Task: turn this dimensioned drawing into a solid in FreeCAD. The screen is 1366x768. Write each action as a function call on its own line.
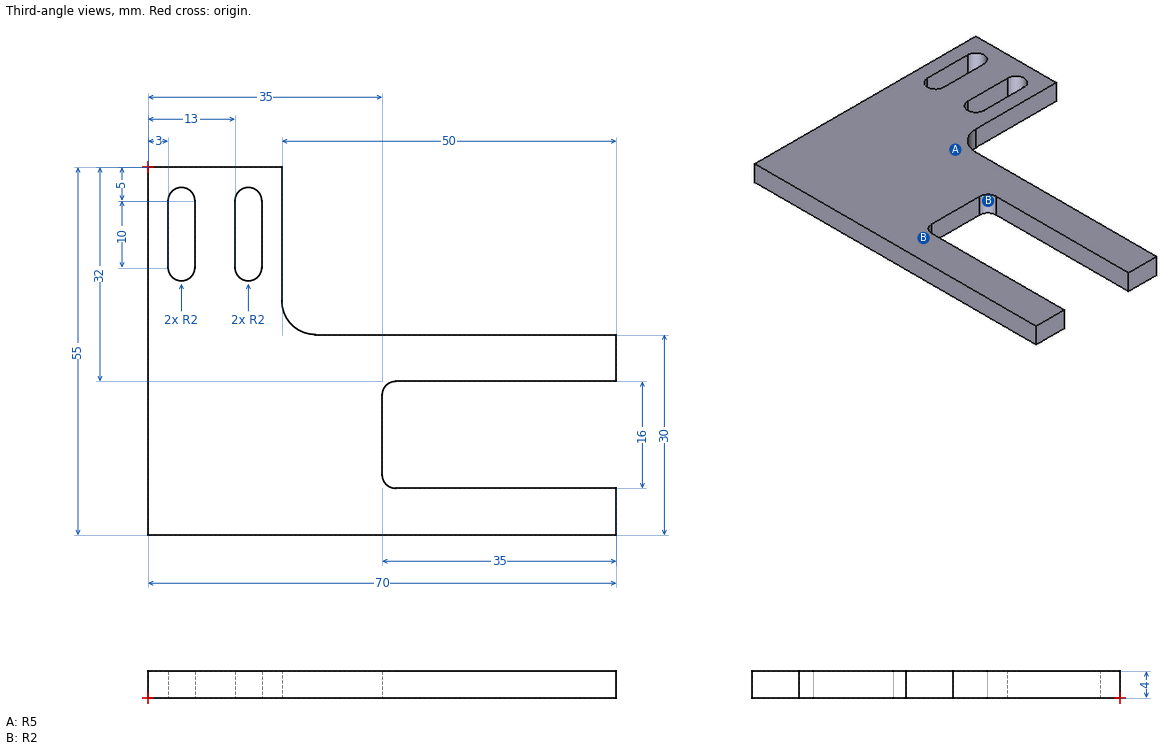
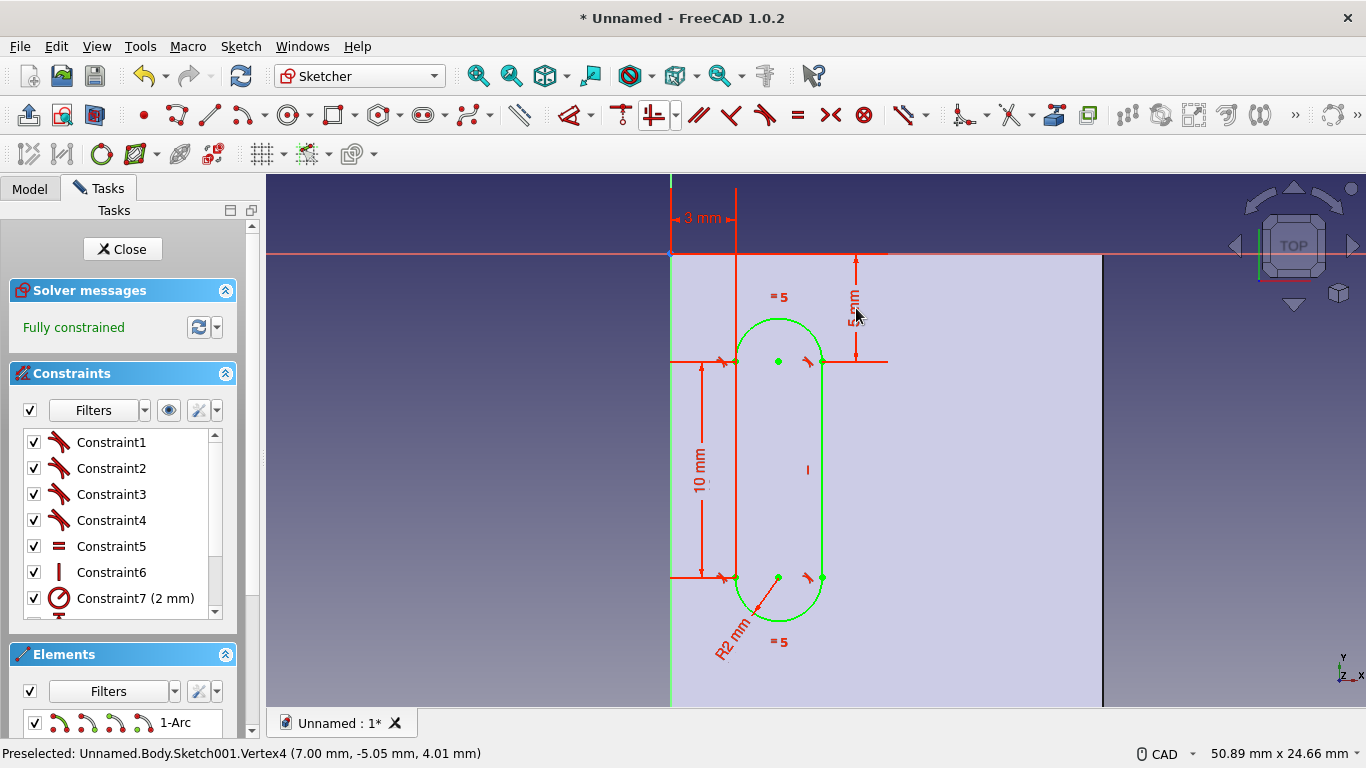
click(123, 249)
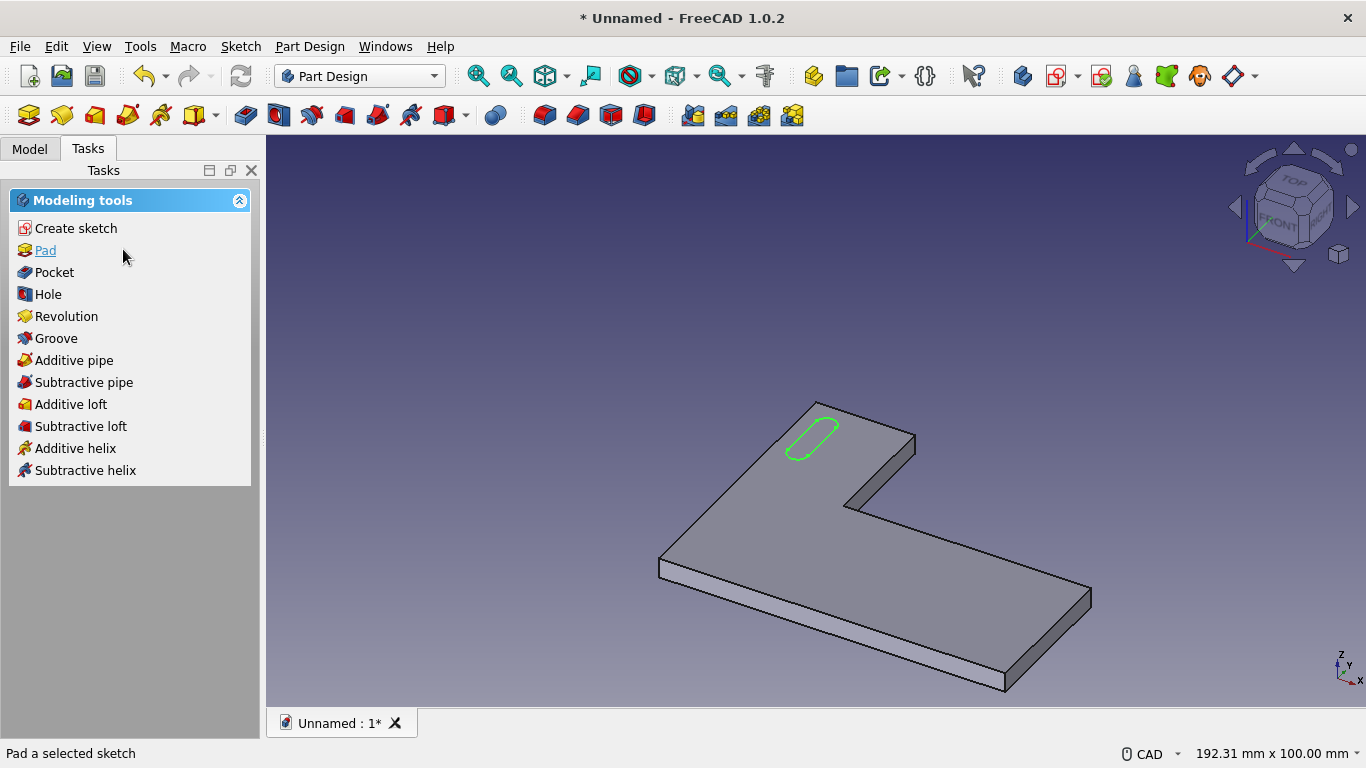
click(246, 116)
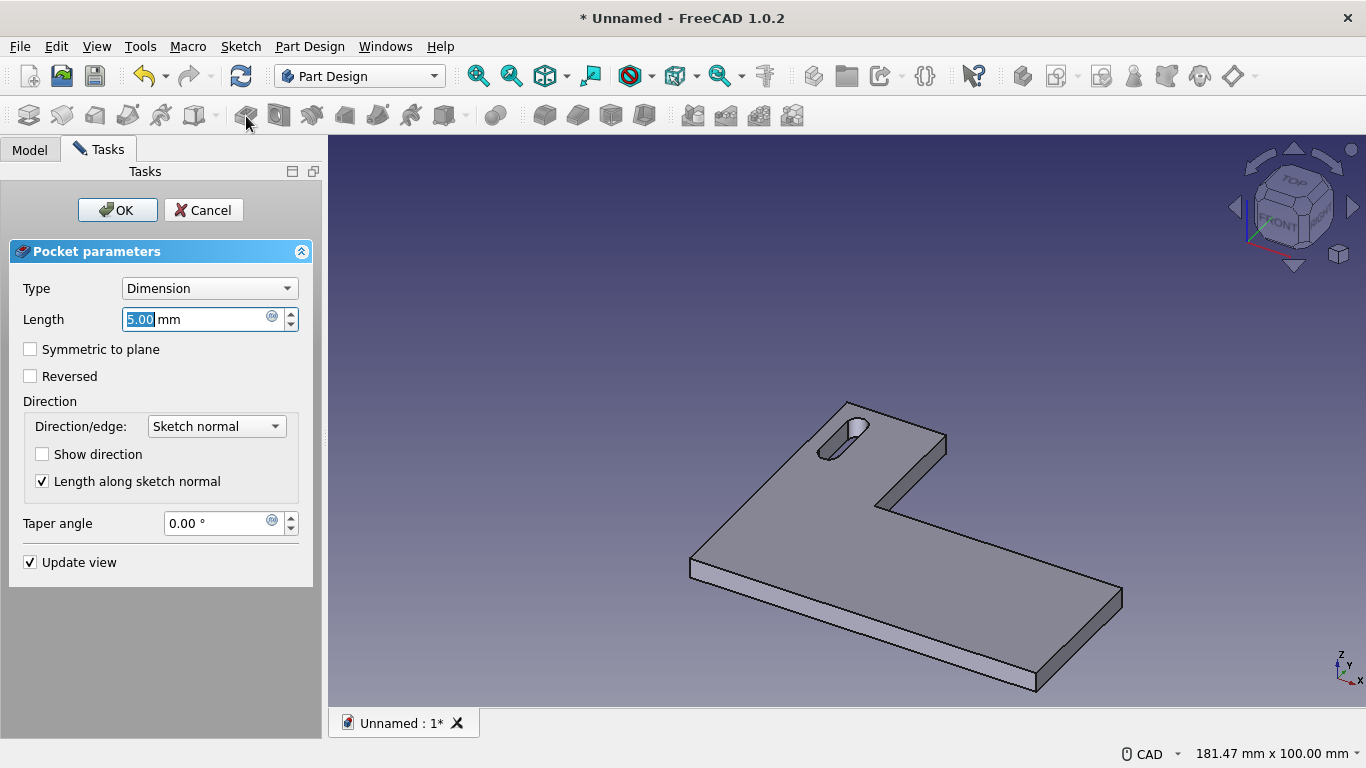
click(210, 288)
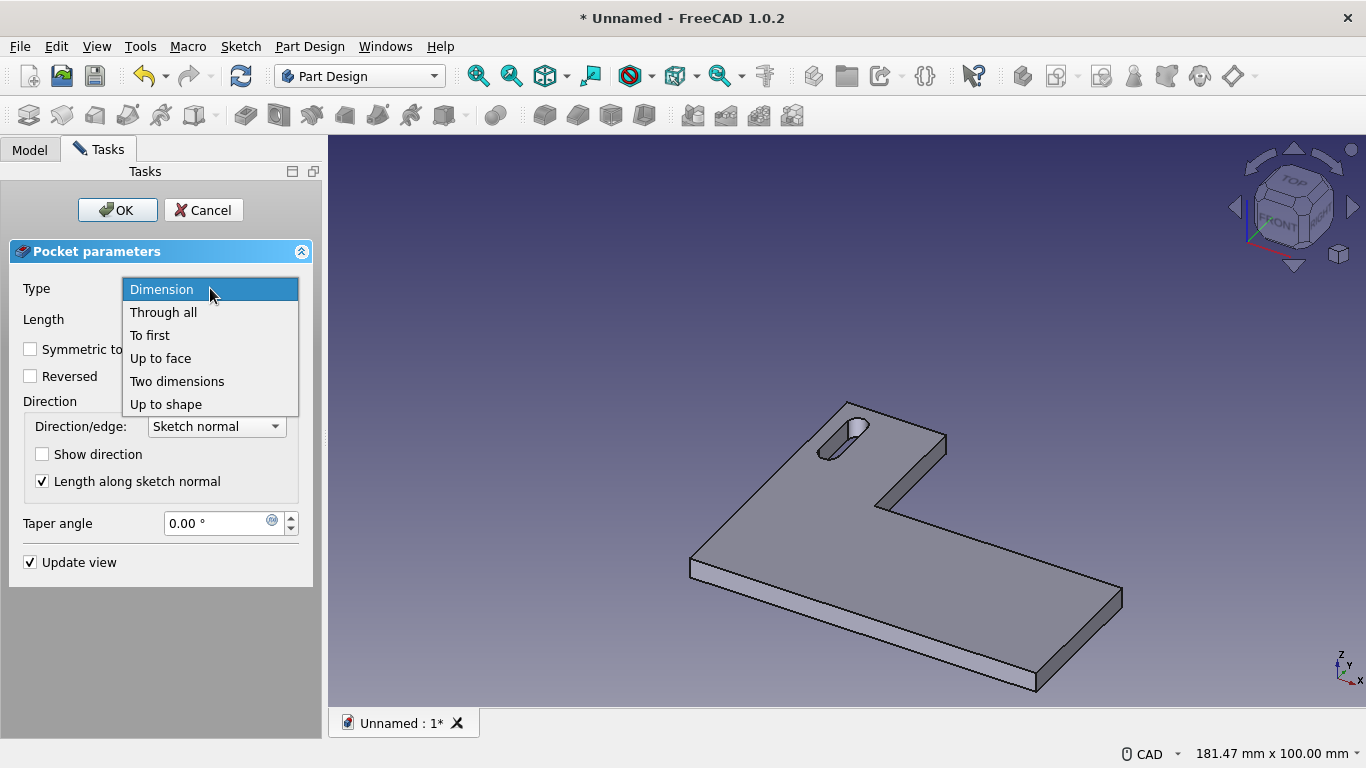
click(208, 336)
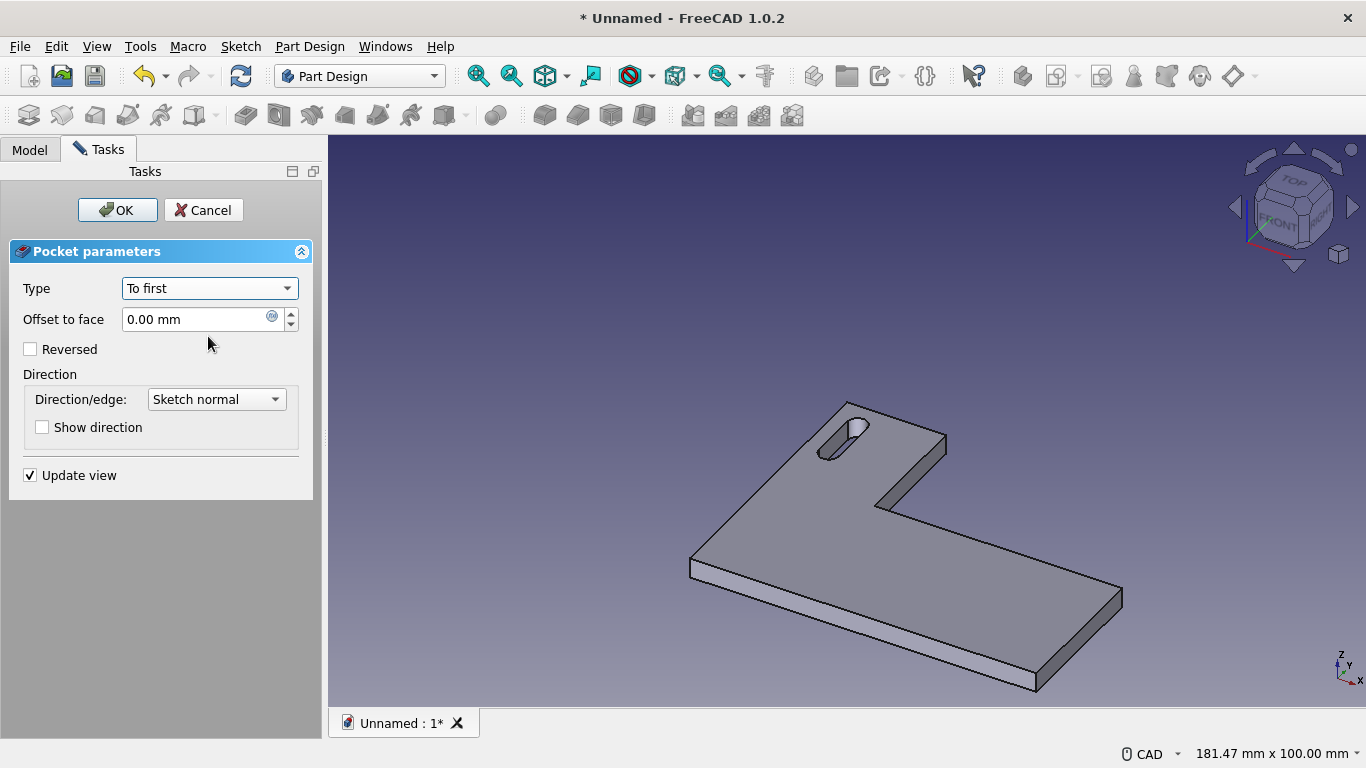
click(118, 210)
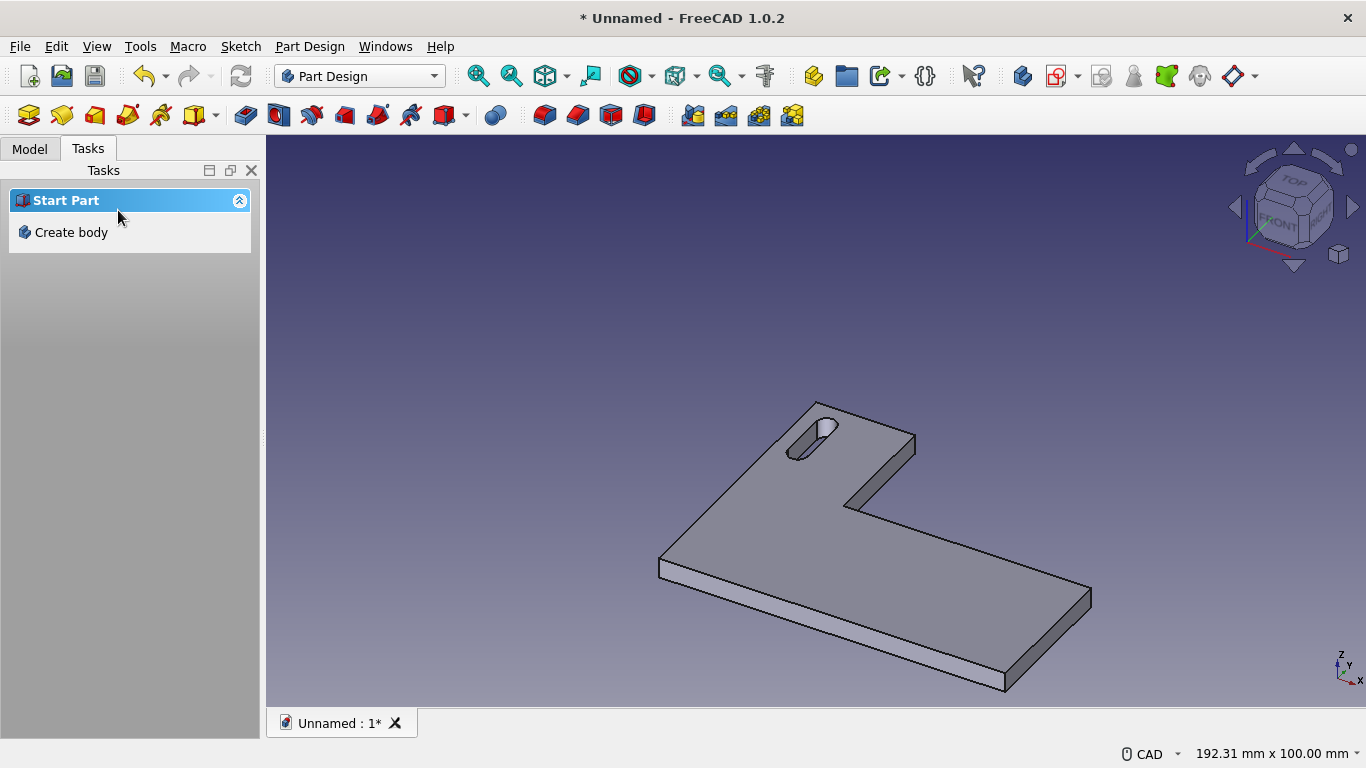
click(965, 614)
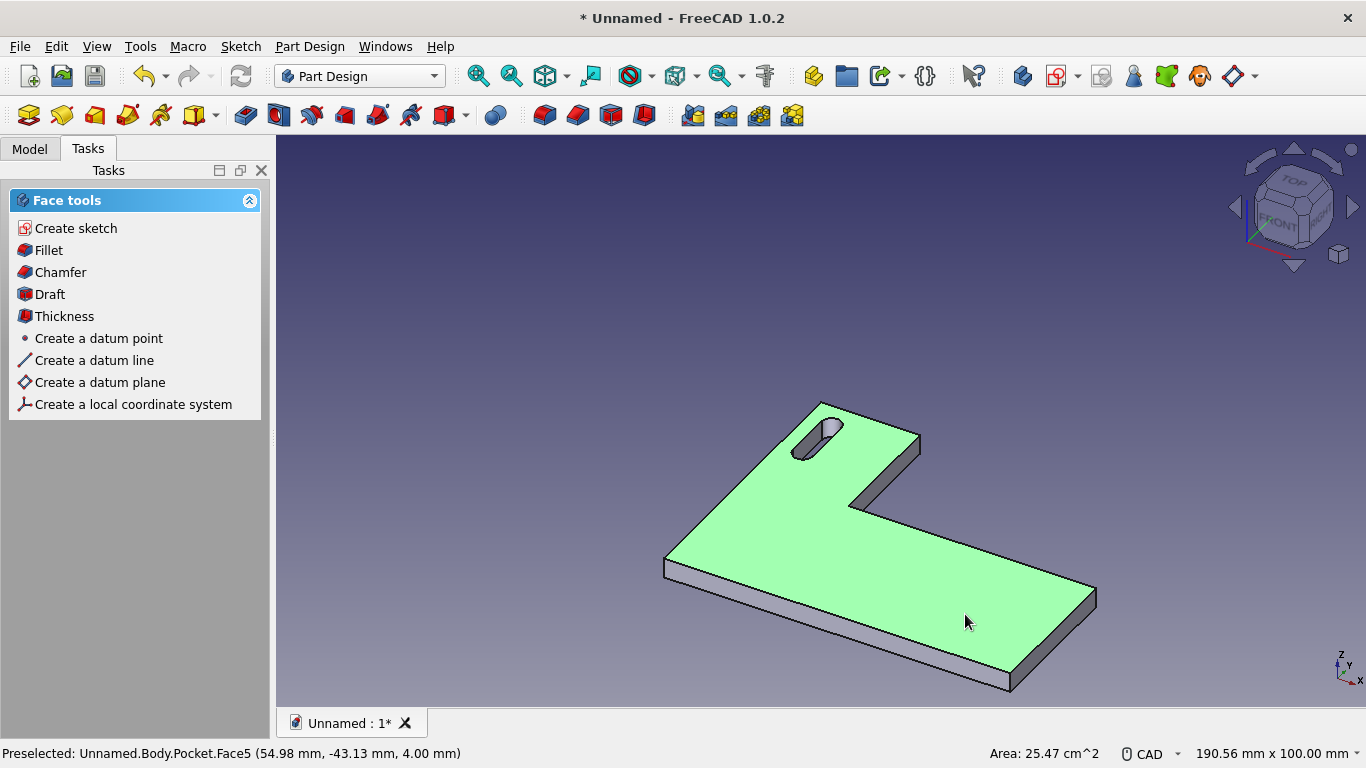
click(1056, 76)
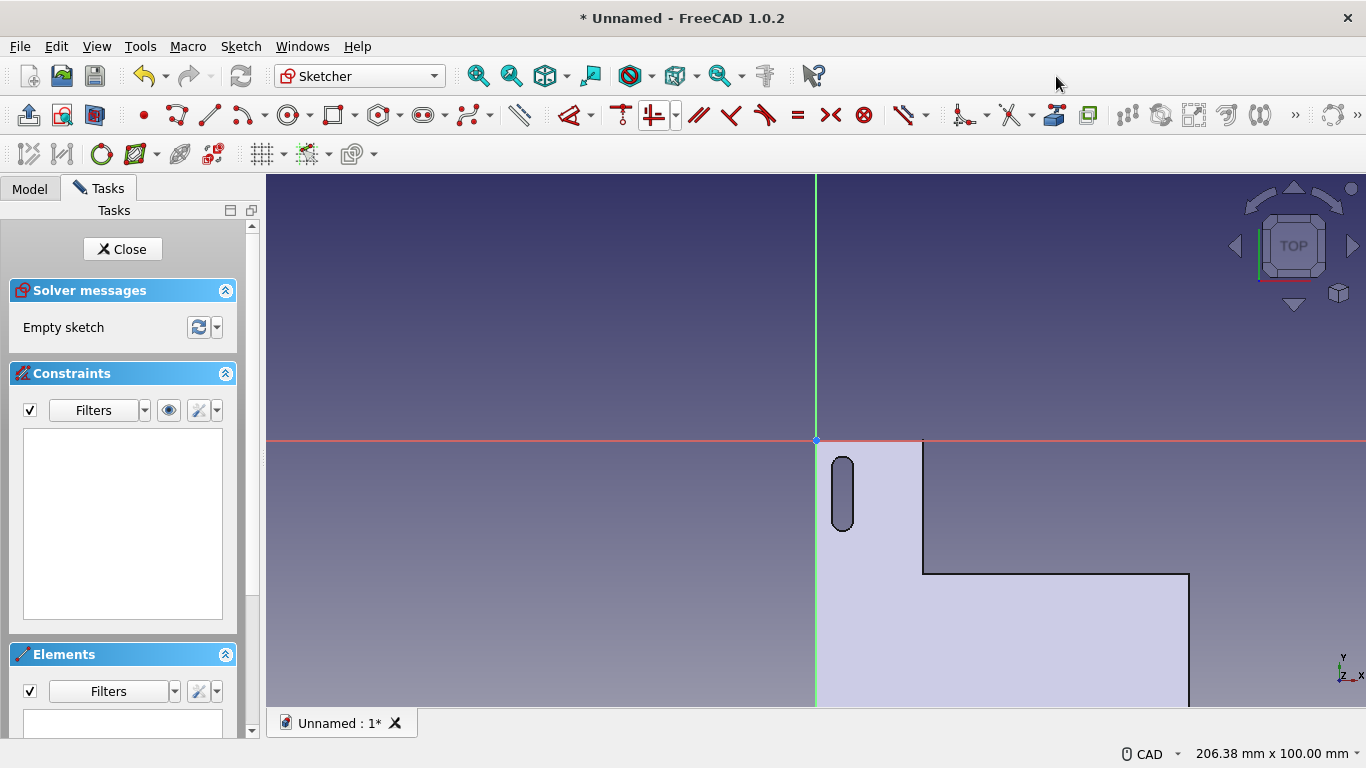
scroll(899, 501, up, 7)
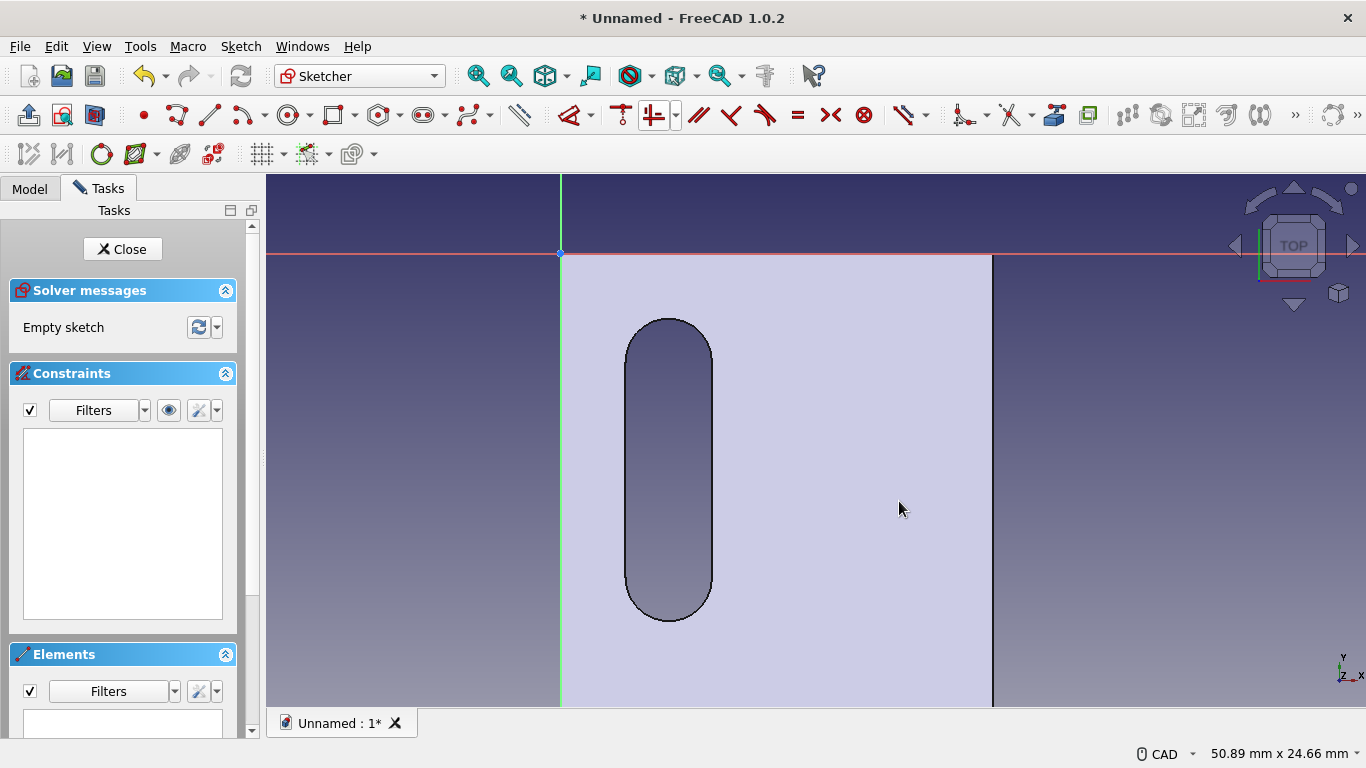
key(g)
key(s)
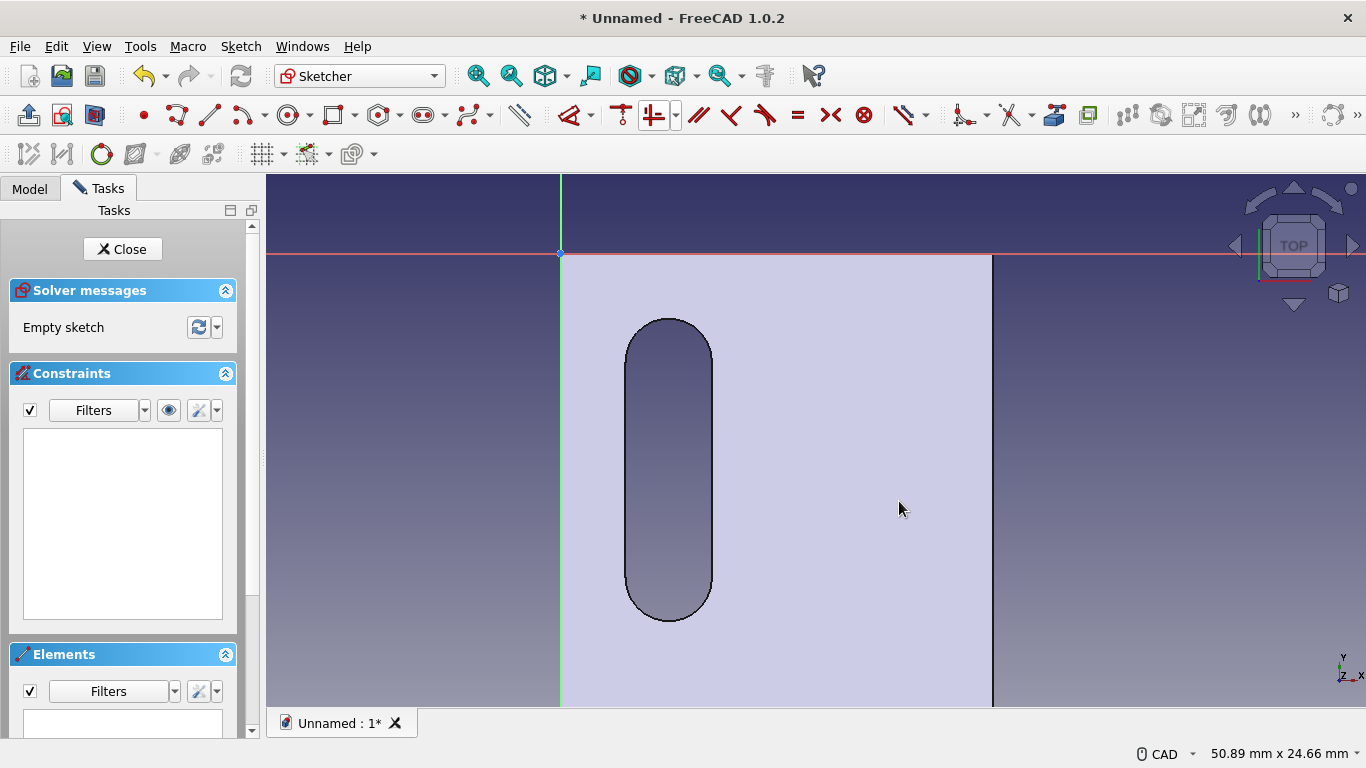
click(885, 578)